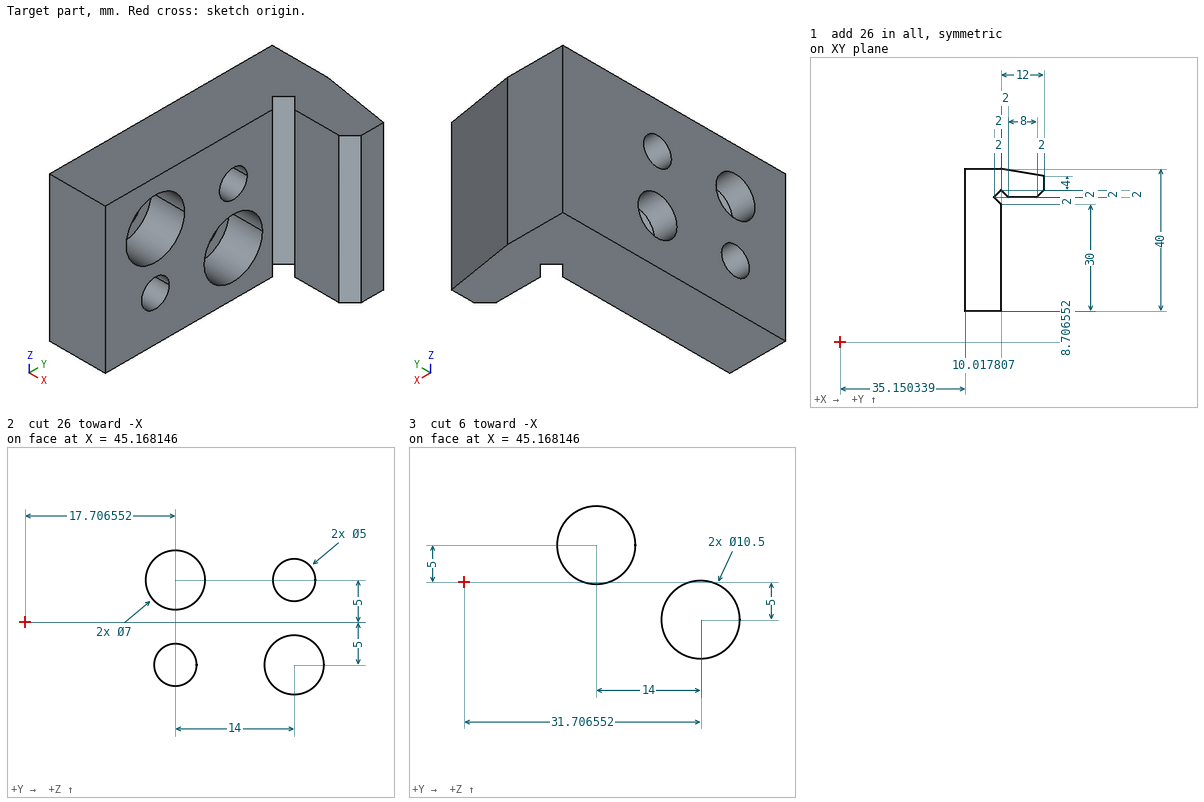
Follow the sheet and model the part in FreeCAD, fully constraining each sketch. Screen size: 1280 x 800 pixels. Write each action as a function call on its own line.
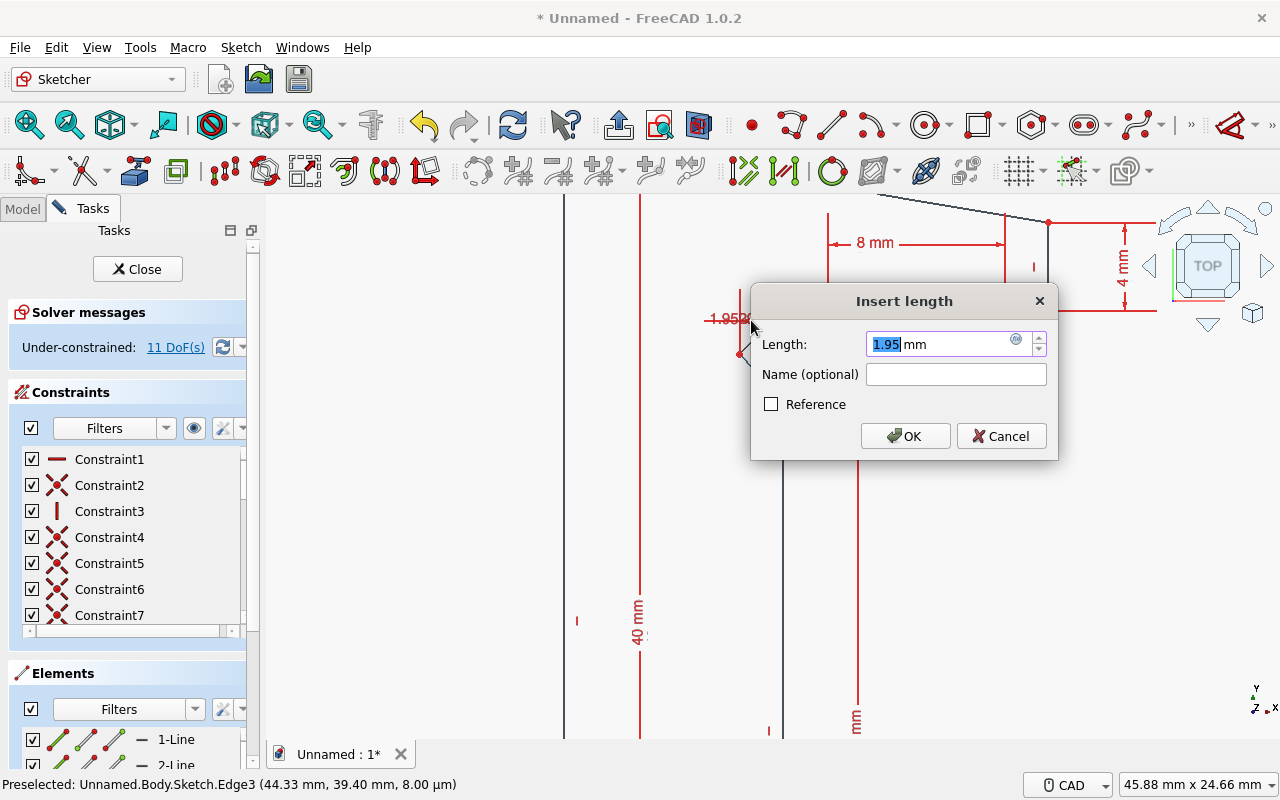
text(2)
key(Return)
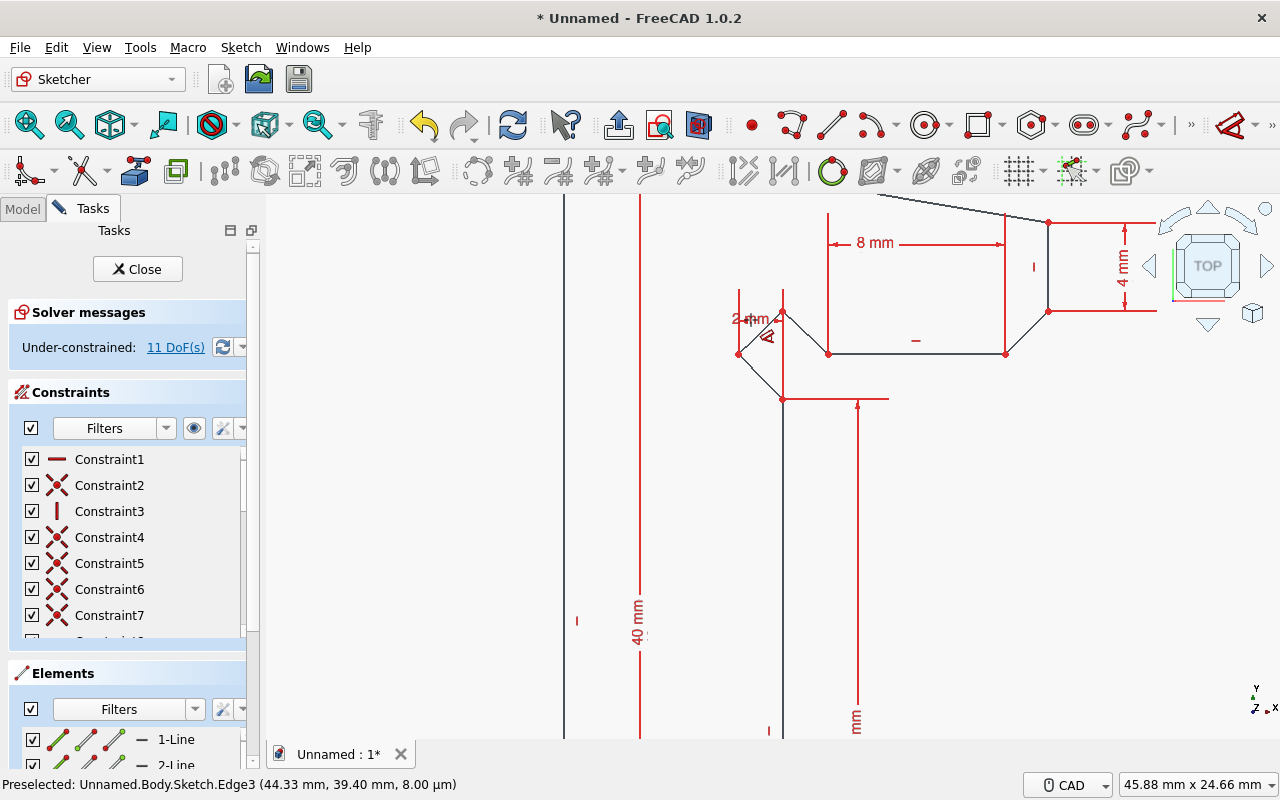
click(769, 386)
click(817, 377)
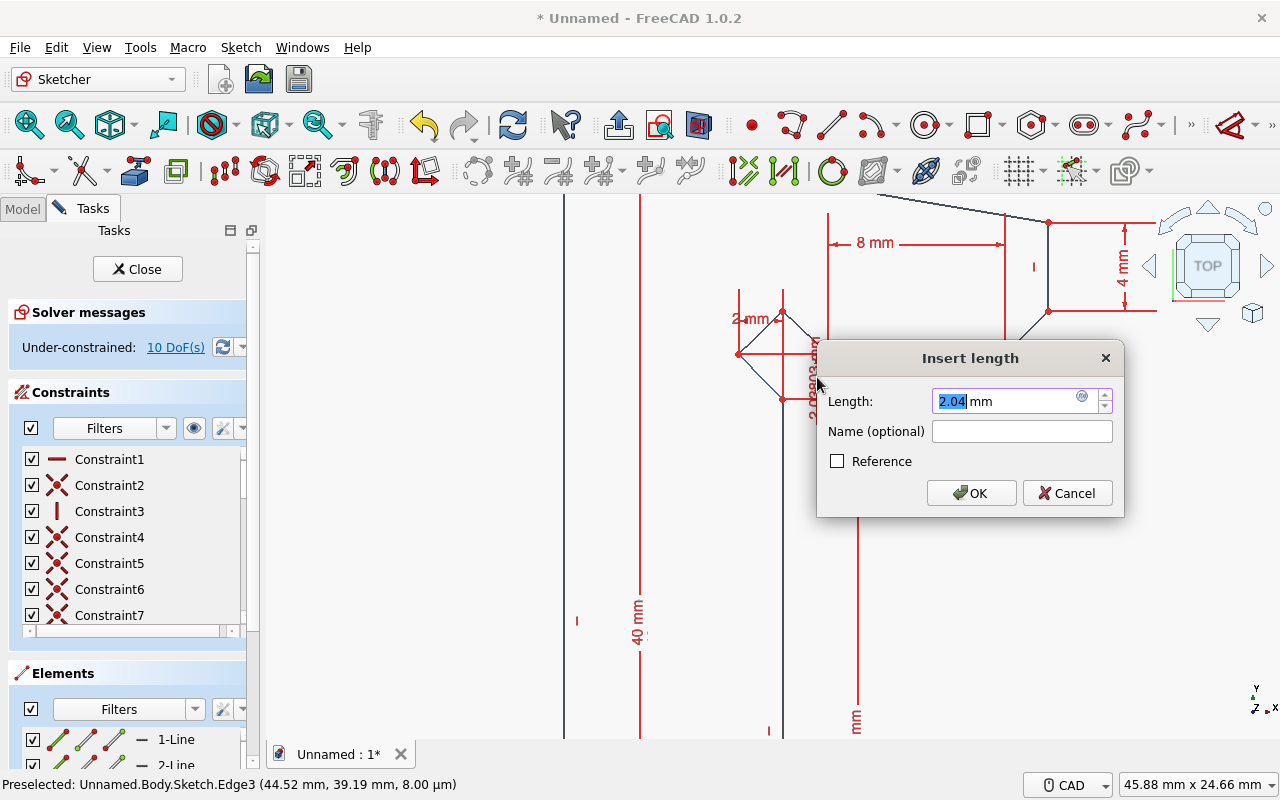
text(2)
key(Return)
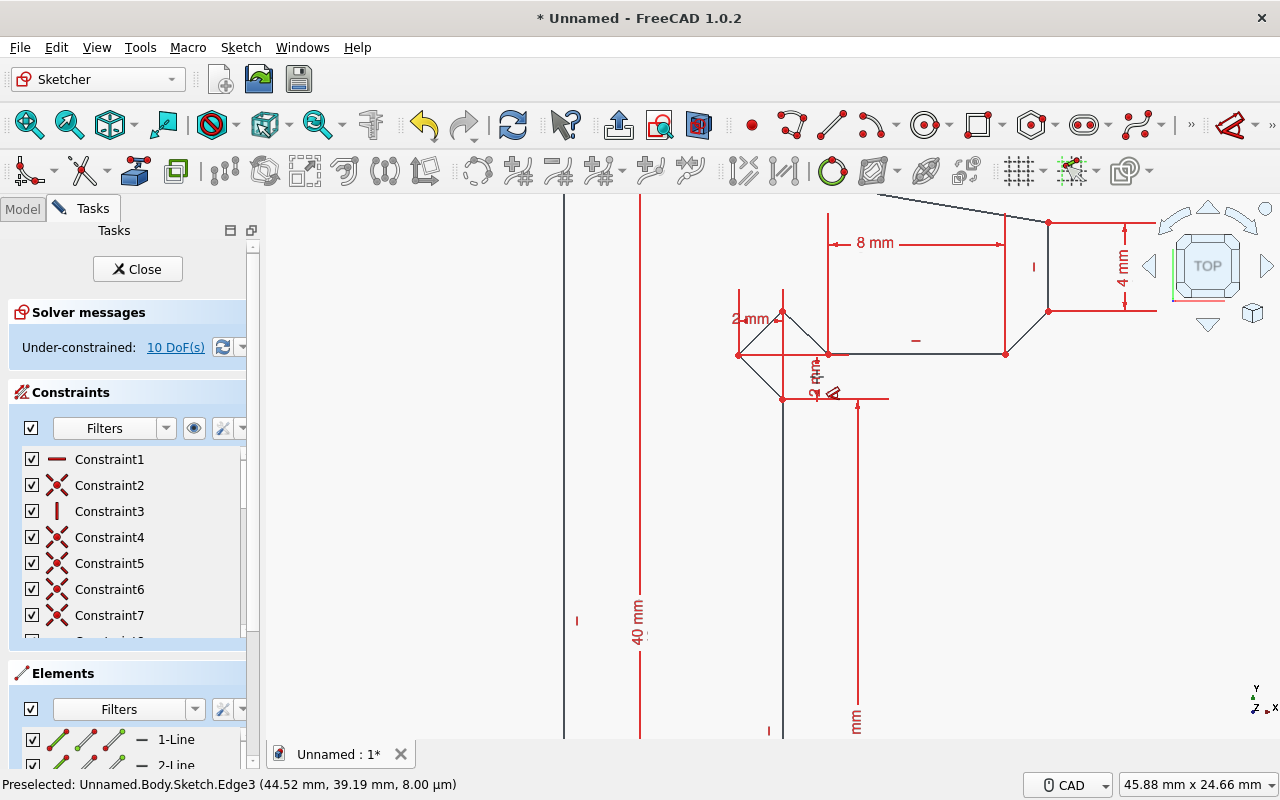
click(752, 342)
click(761, 277)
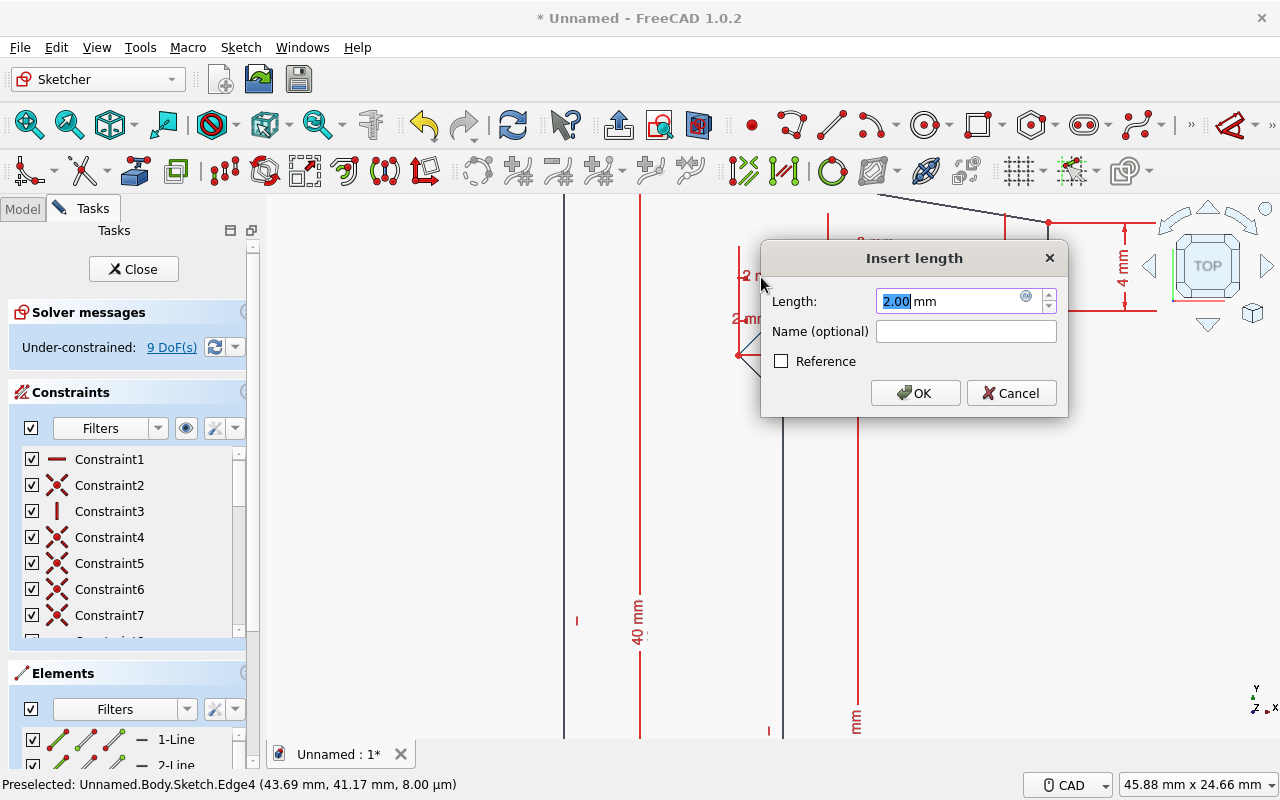
text(2)
key(Return)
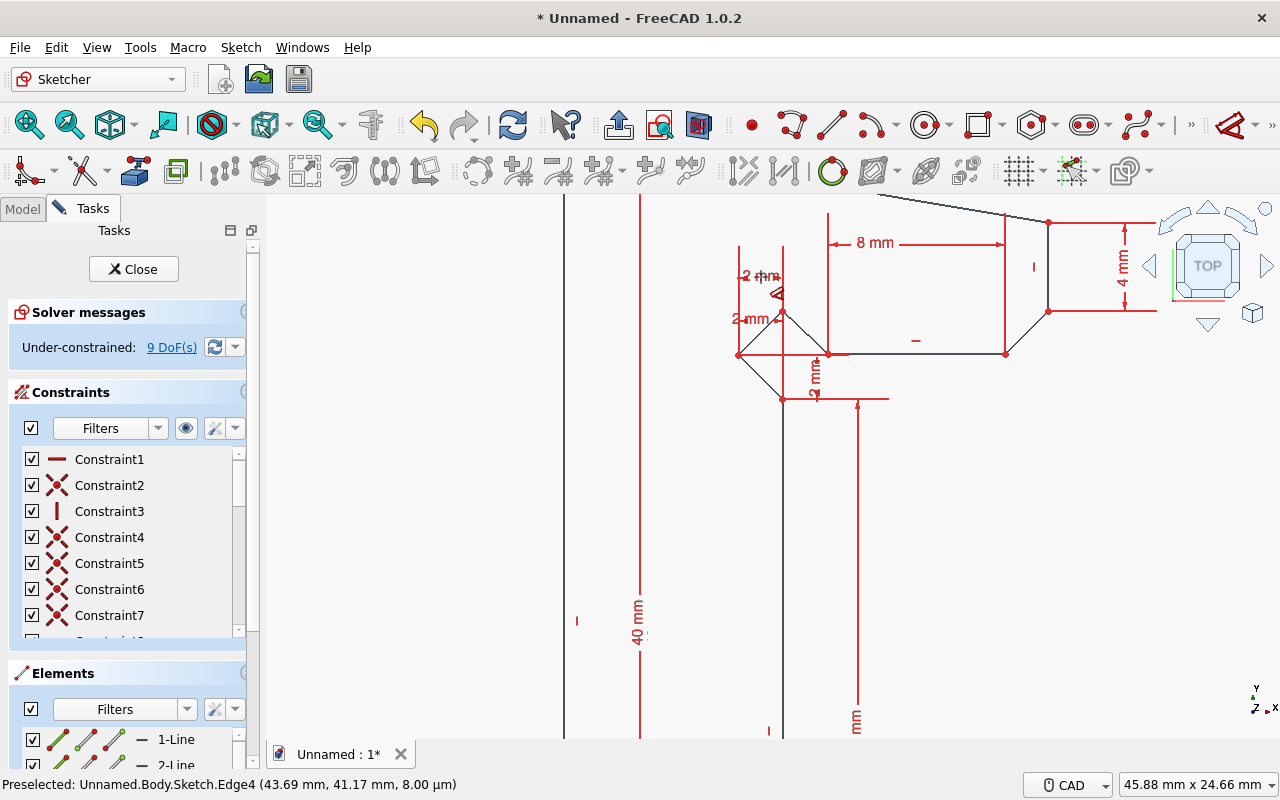
click(752, 342)
click(705, 343)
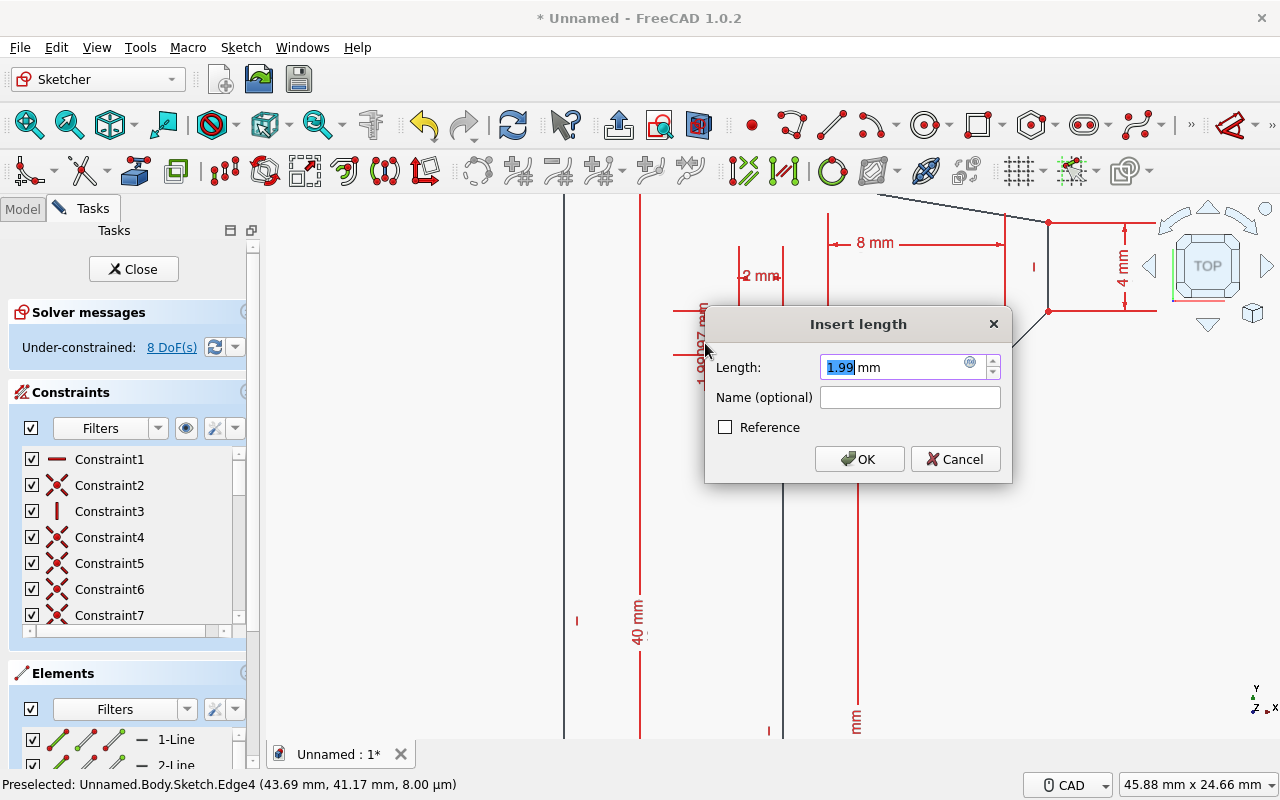
text(2)
key(Return)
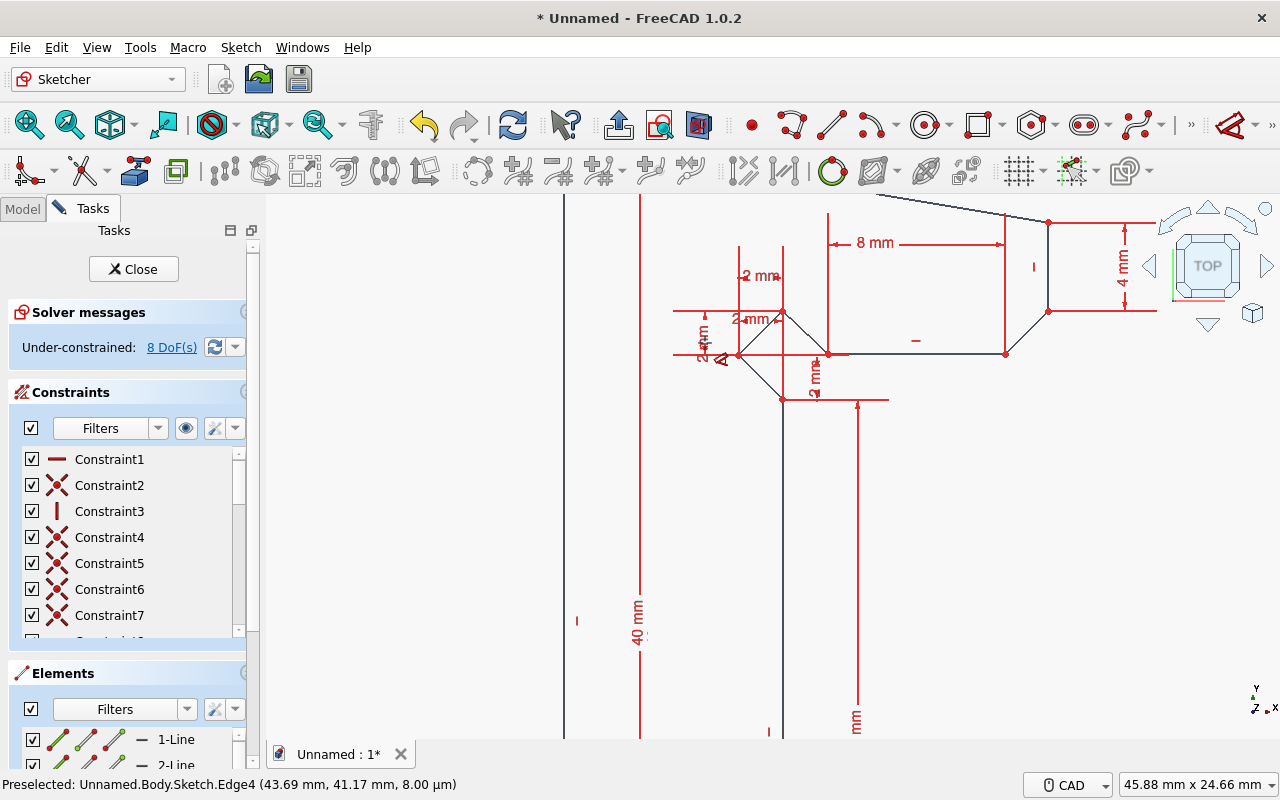
click(796, 324)
click(806, 253)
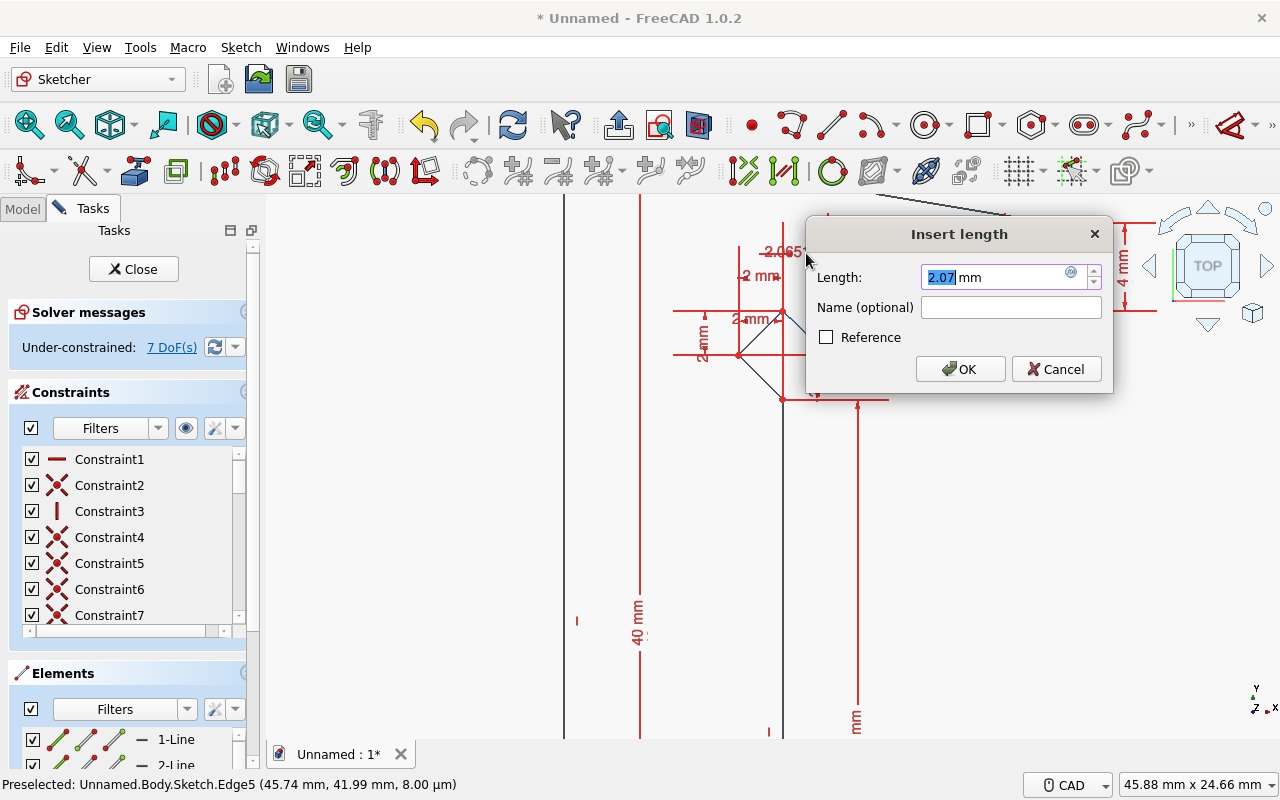
text(2)
key(Return)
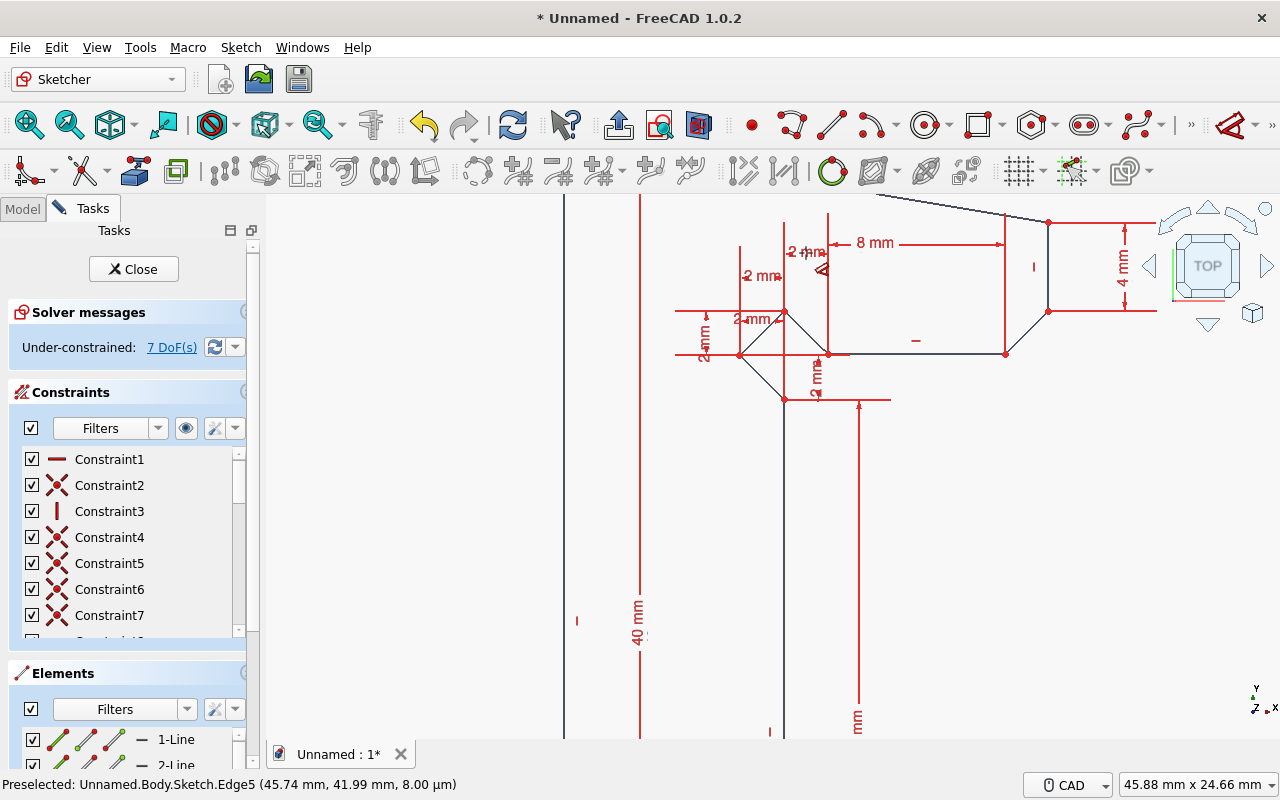
click(797, 324)
click(862, 333)